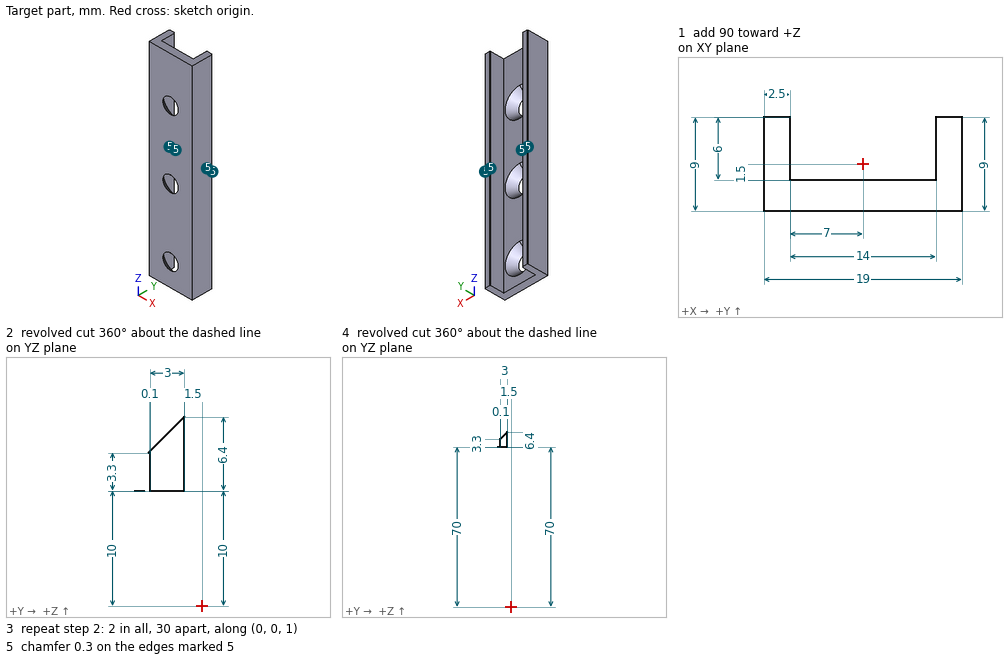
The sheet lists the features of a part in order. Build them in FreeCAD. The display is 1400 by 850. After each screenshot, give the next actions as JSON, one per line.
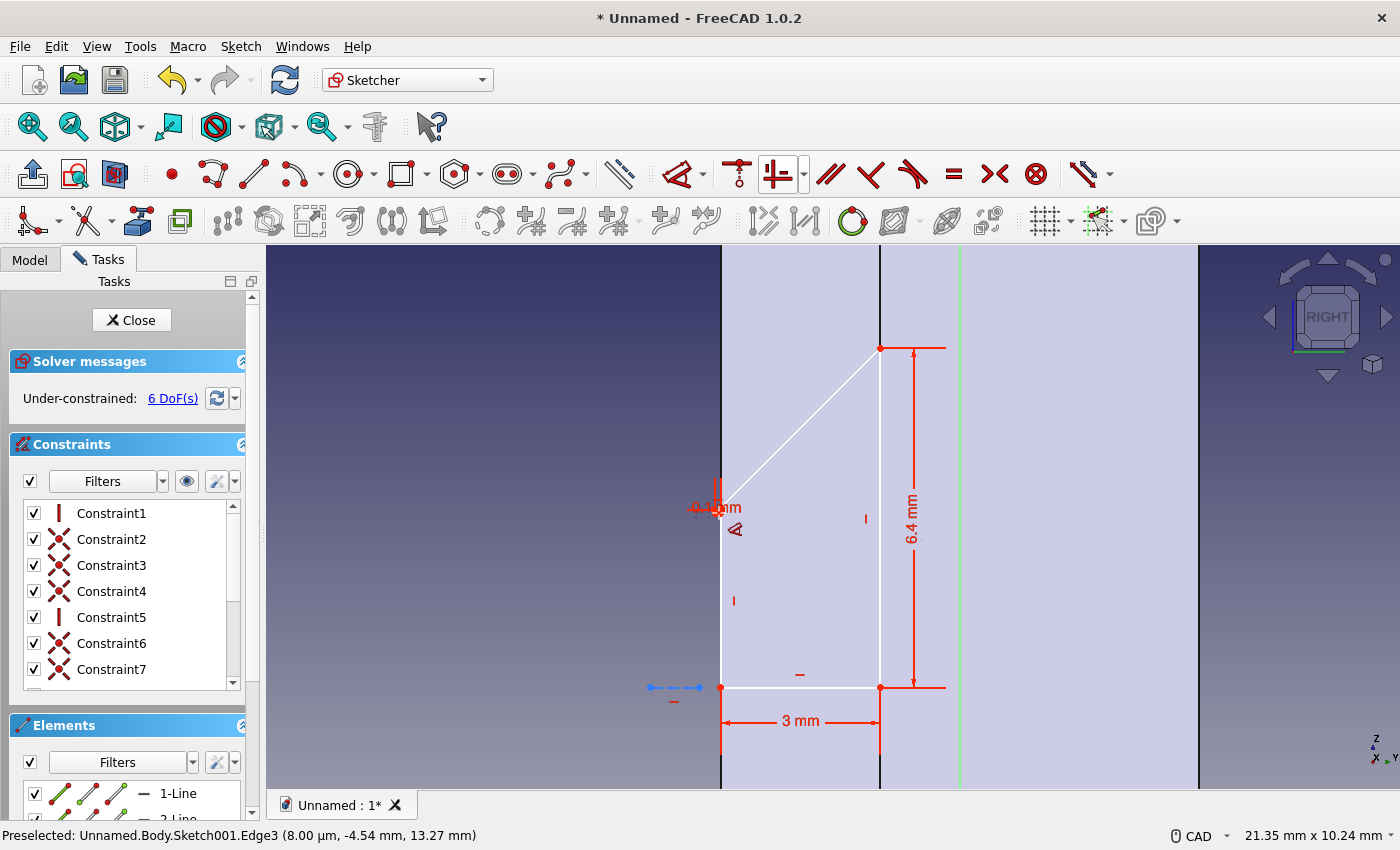
{"action": "left_click", "coordinate": [721, 566]}
{"action": "left_click", "coordinate": [687, 601]}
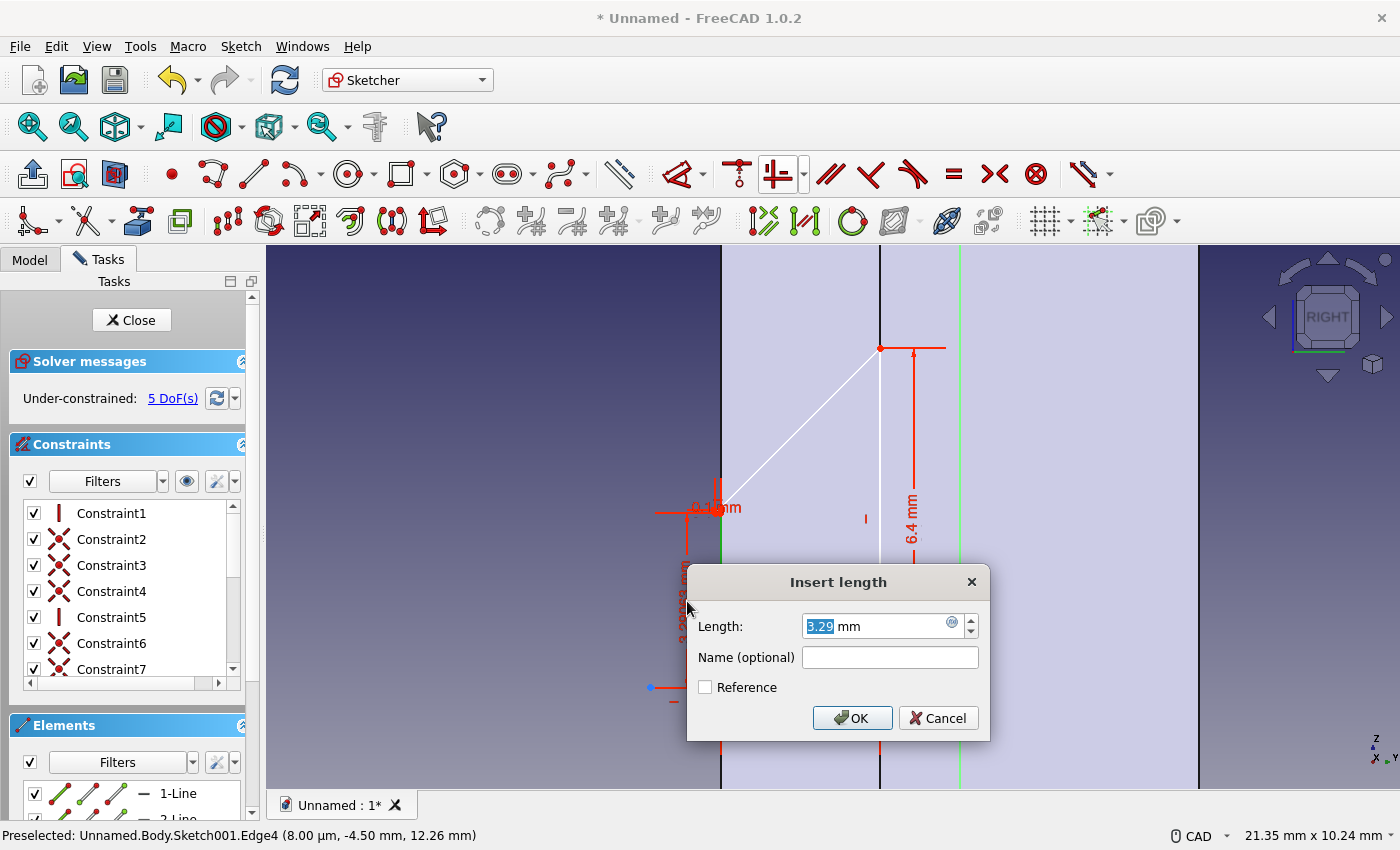
{"action": "type", "text": "3.3"}
{"action": "key", "text": "Return"}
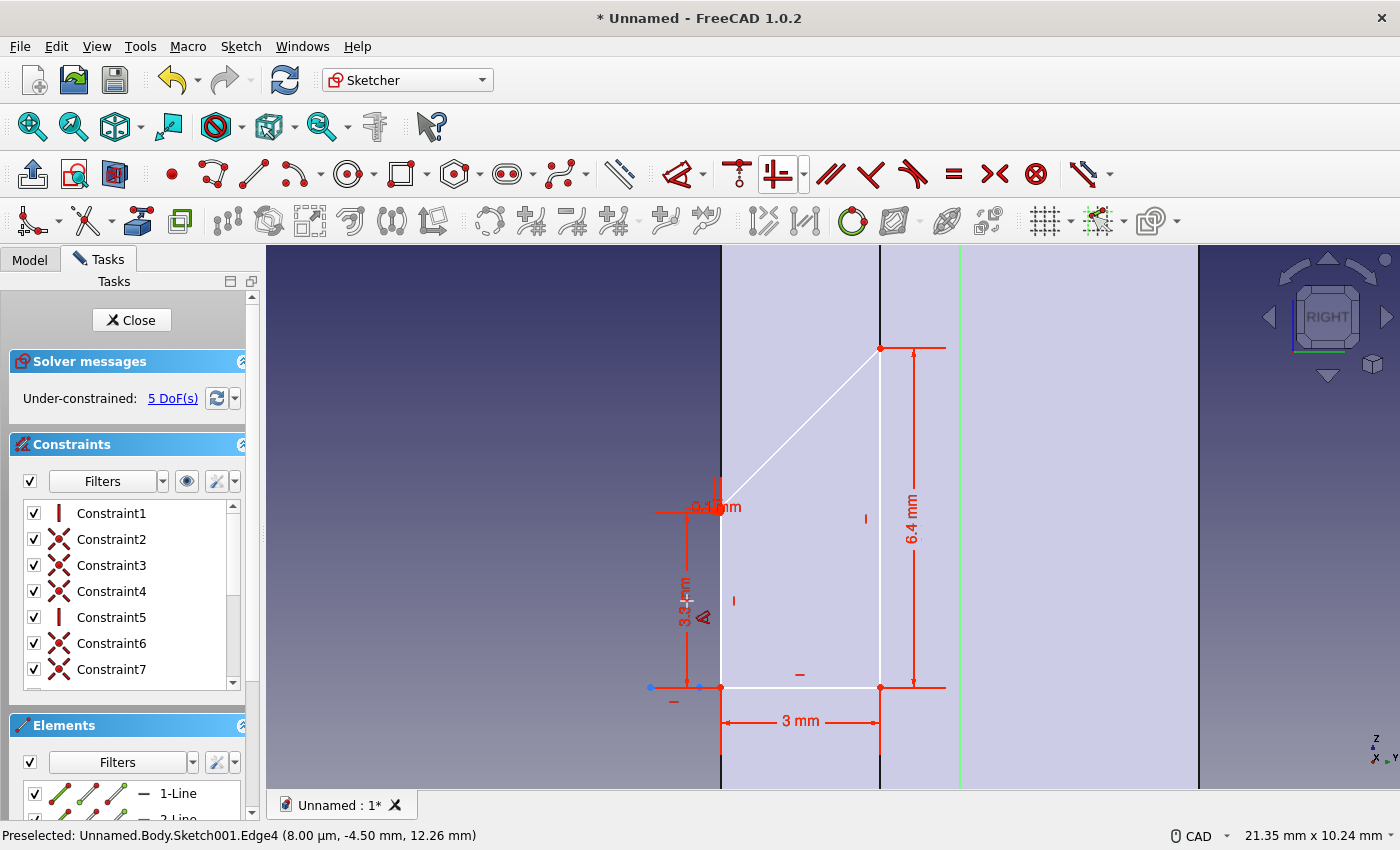
{"action": "left_click", "coordinate": [880, 688]}
{"action": "left_click", "coordinate": [994, 724]}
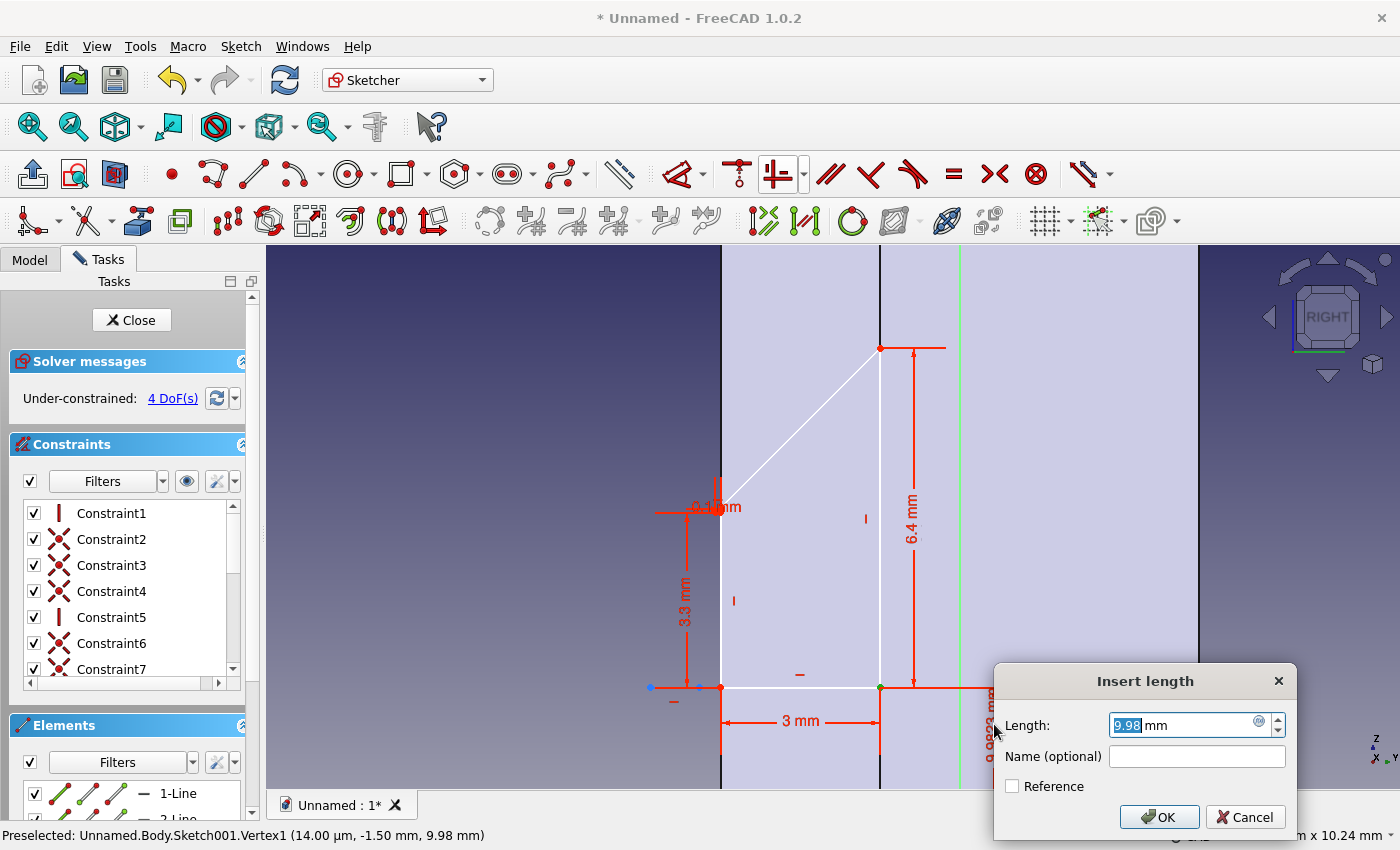
{"action": "type", "text": "10"}
{"action": "key", "text": "Return"}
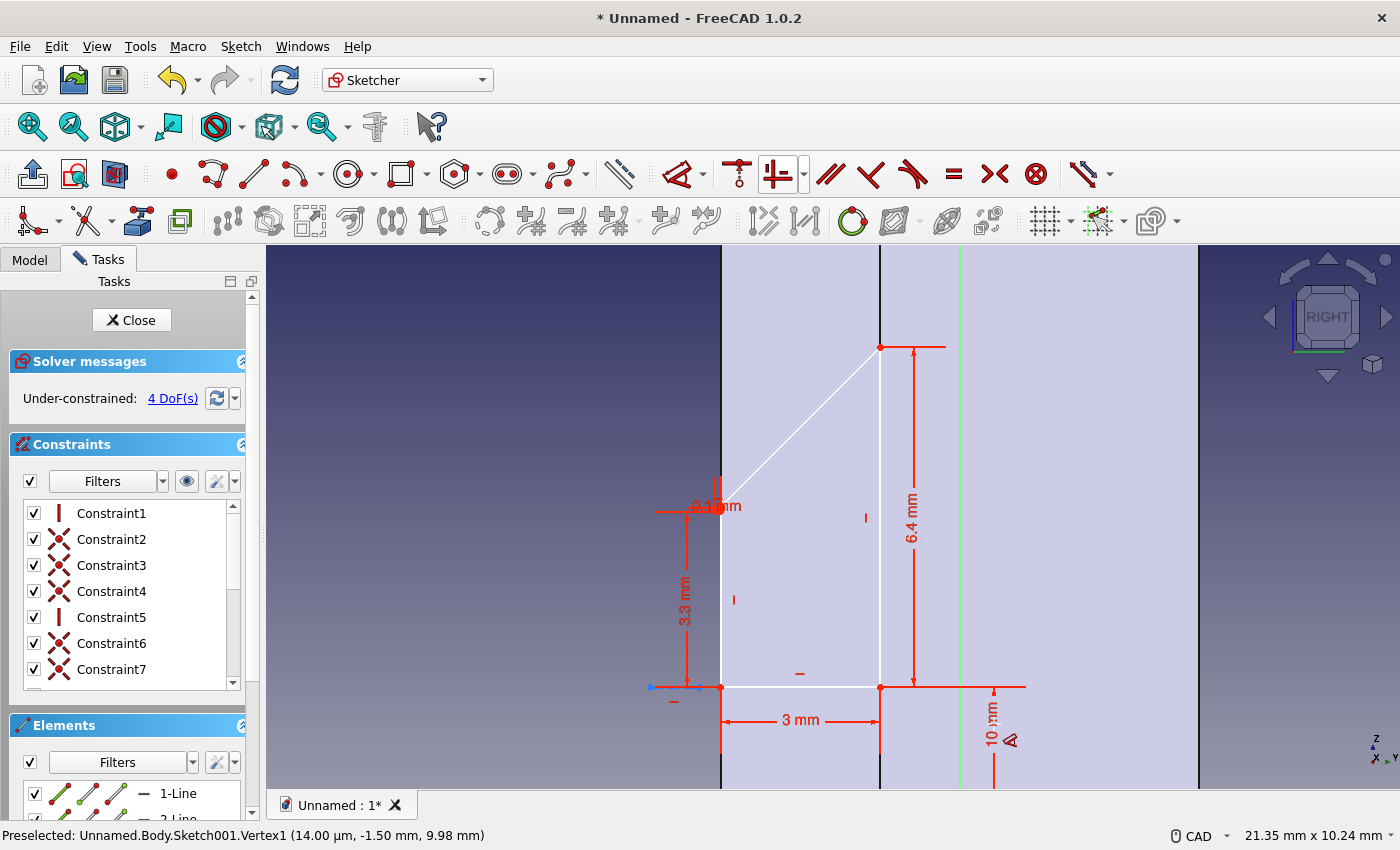
{"action": "left_click", "coordinate": [699, 688]}
{"action": "left_click", "coordinate": [994, 699]}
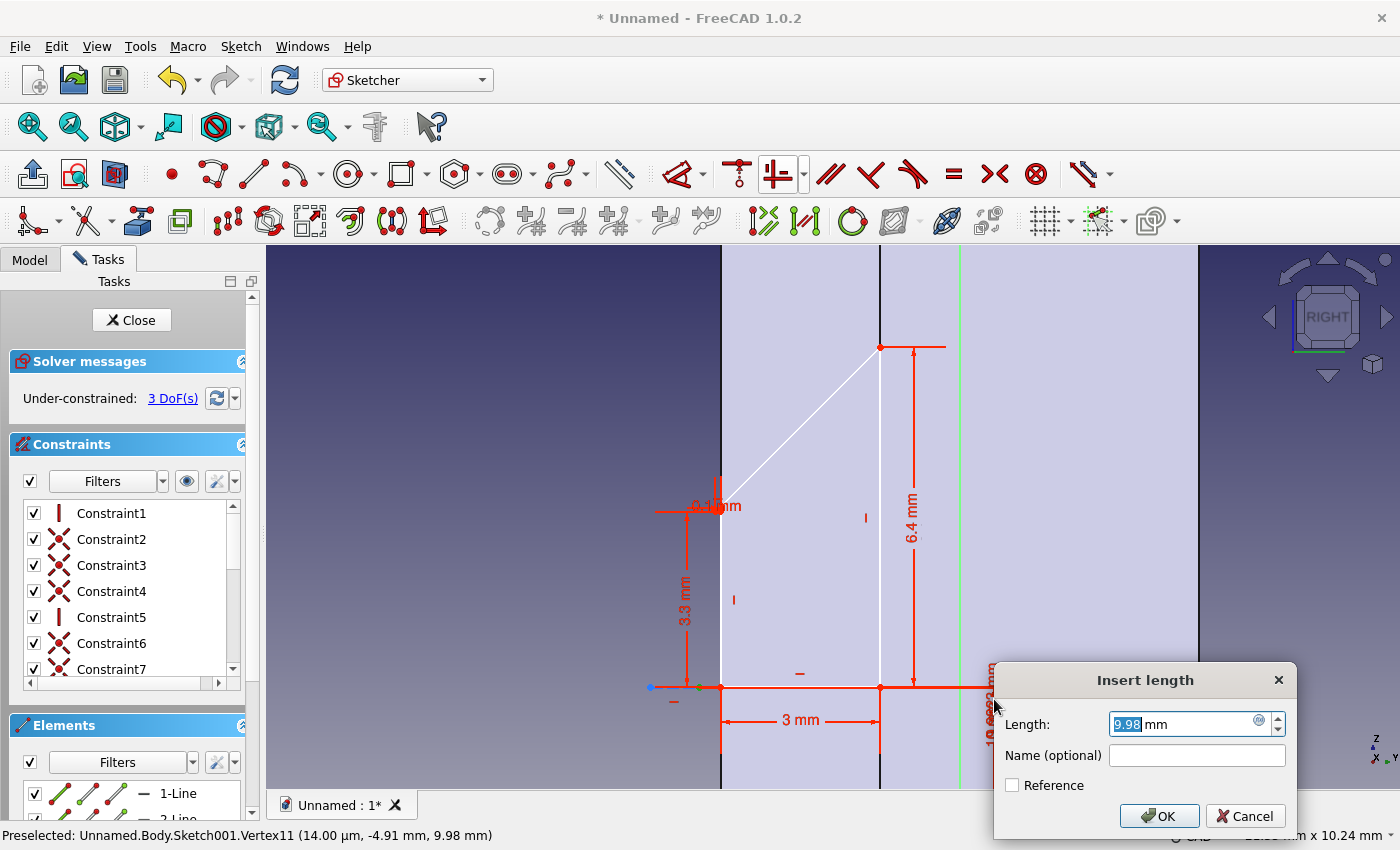
{"action": "type", "text": "10"}
{"action": "key", "text": "Return"}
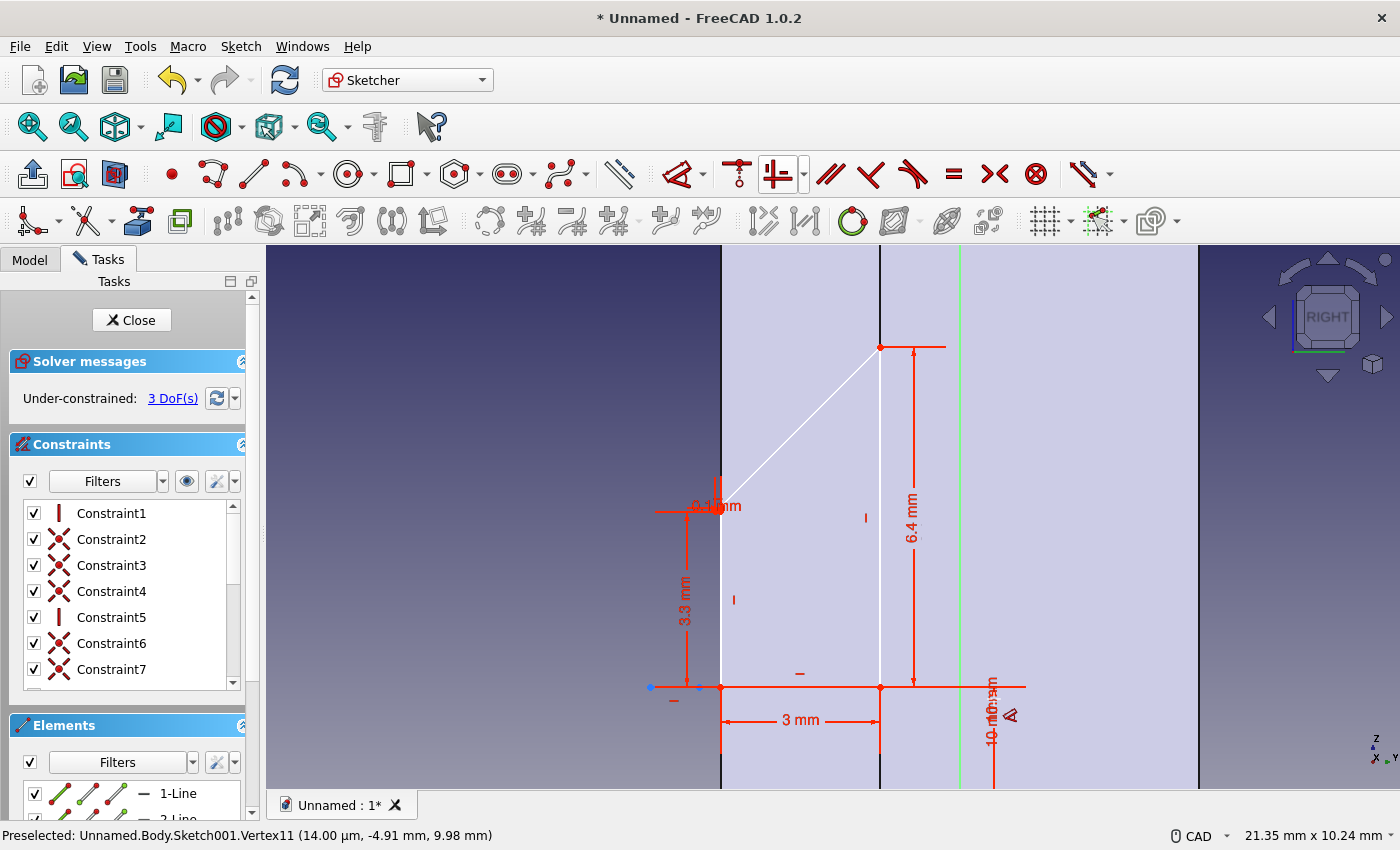
{"action": "left_click", "coordinate": [880, 687]}
{"action": "left_click", "coordinate": [920, 653]}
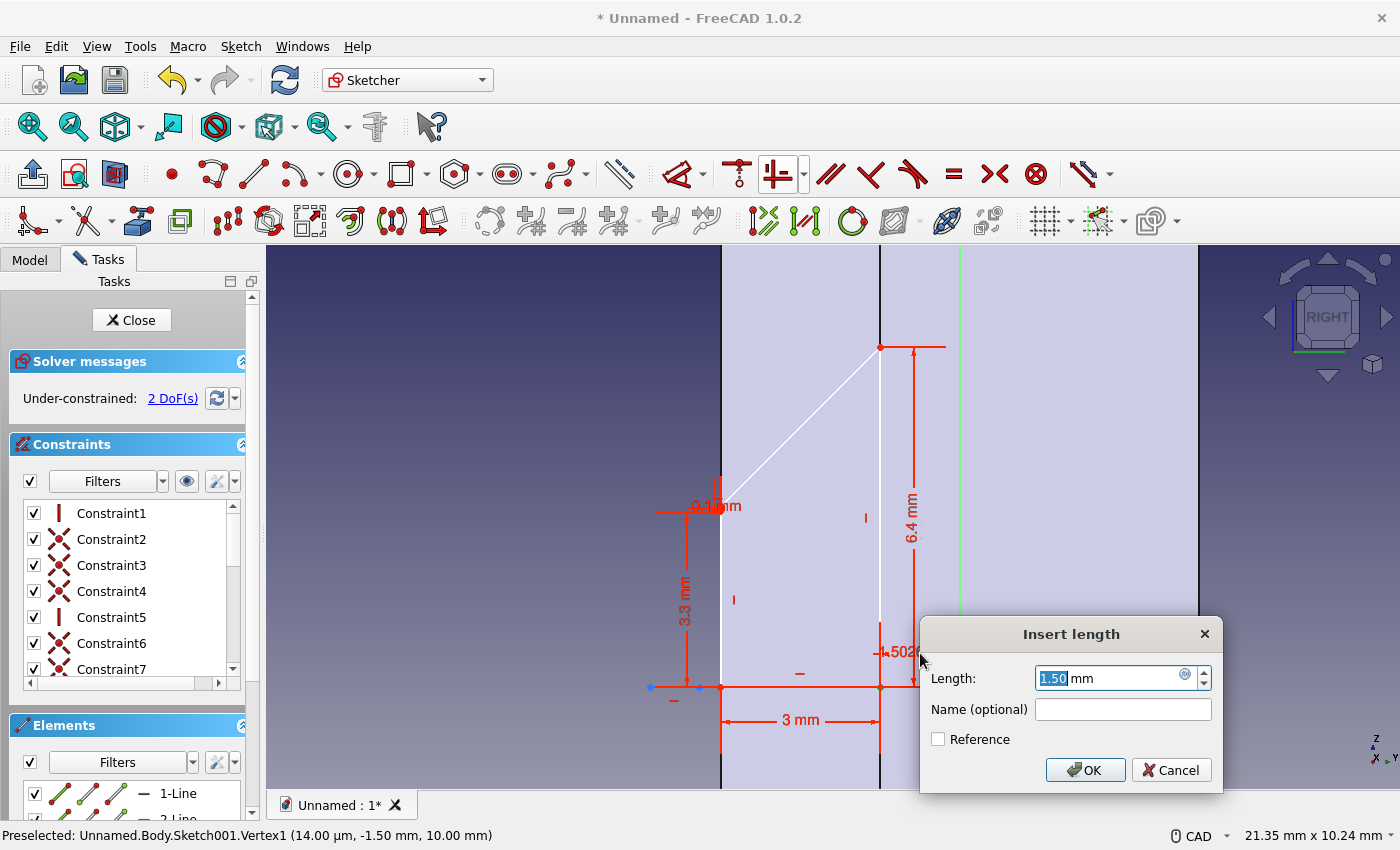
{"action": "type", "text": "1.5"}
{"action": "key", "text": "Return"}
{"action": "key", "text": "Escape"}